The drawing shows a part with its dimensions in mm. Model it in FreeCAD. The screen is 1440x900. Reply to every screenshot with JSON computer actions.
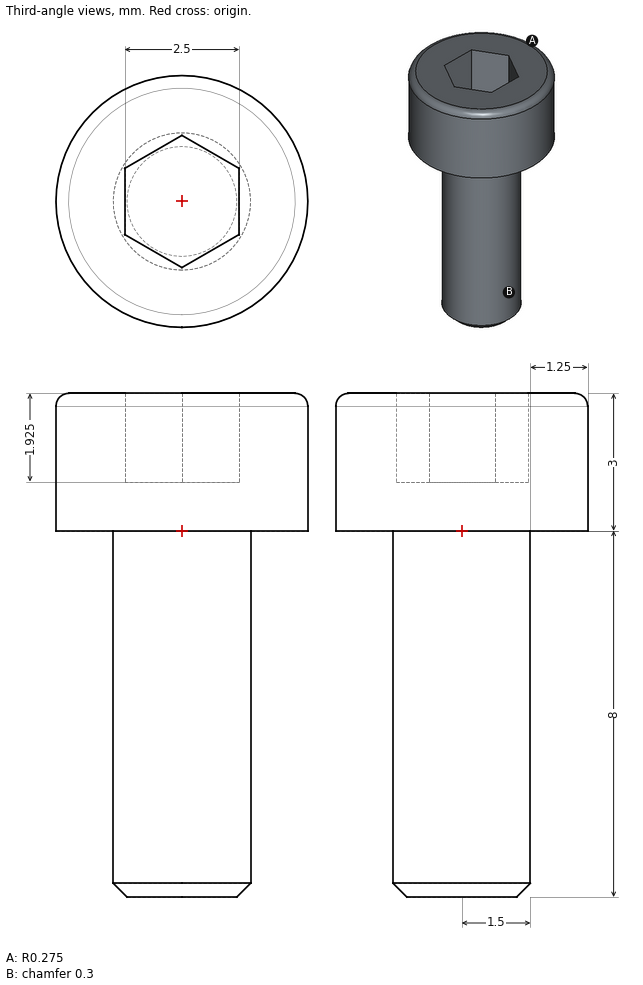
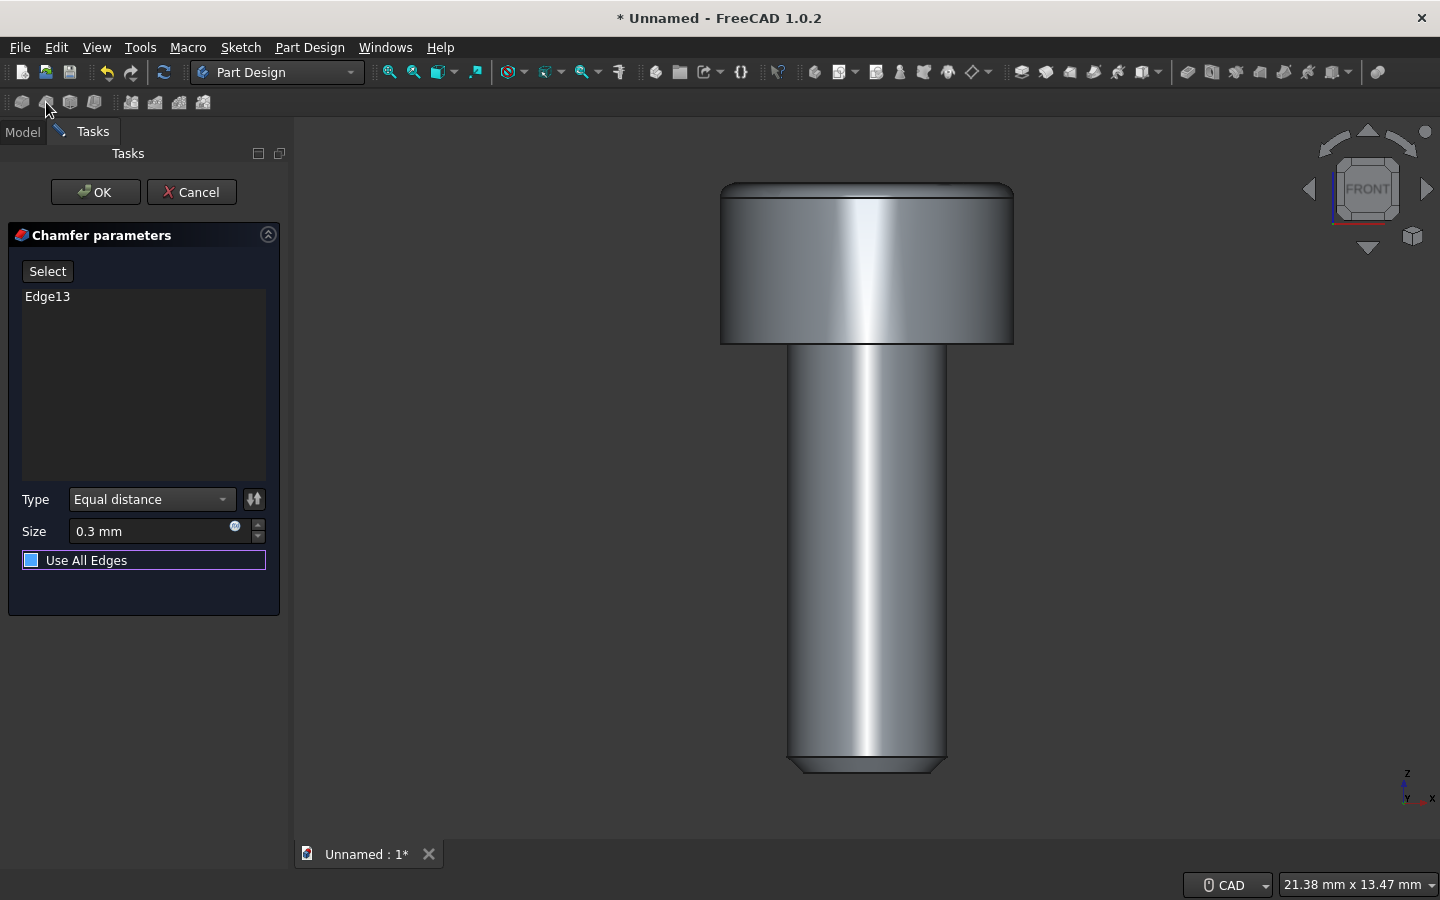
{"action": "left_click", "coordinate": [96, 192]}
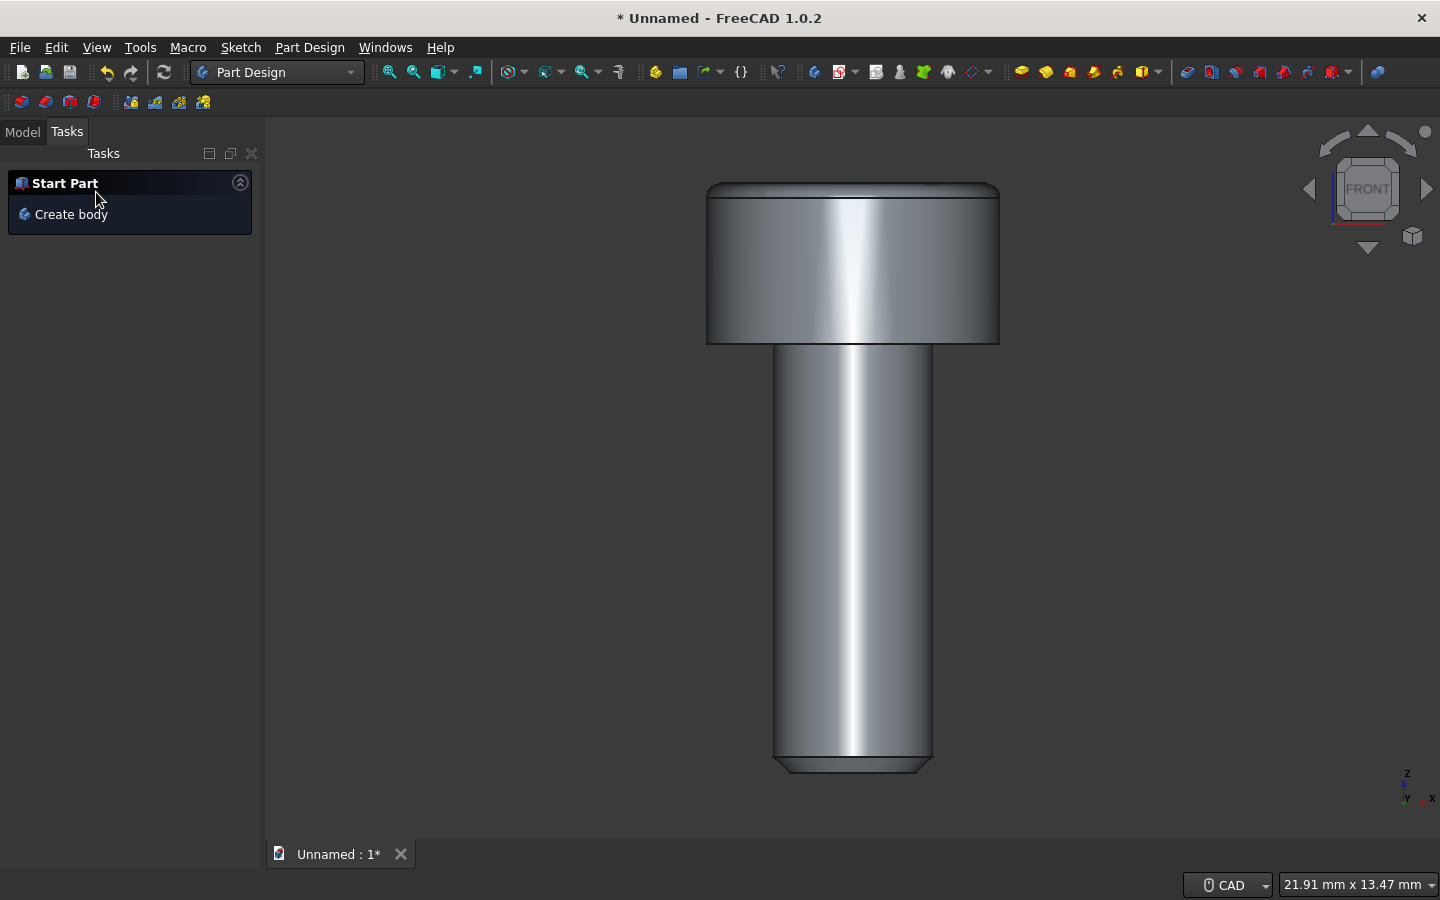
{"action": "key", "text": "0"}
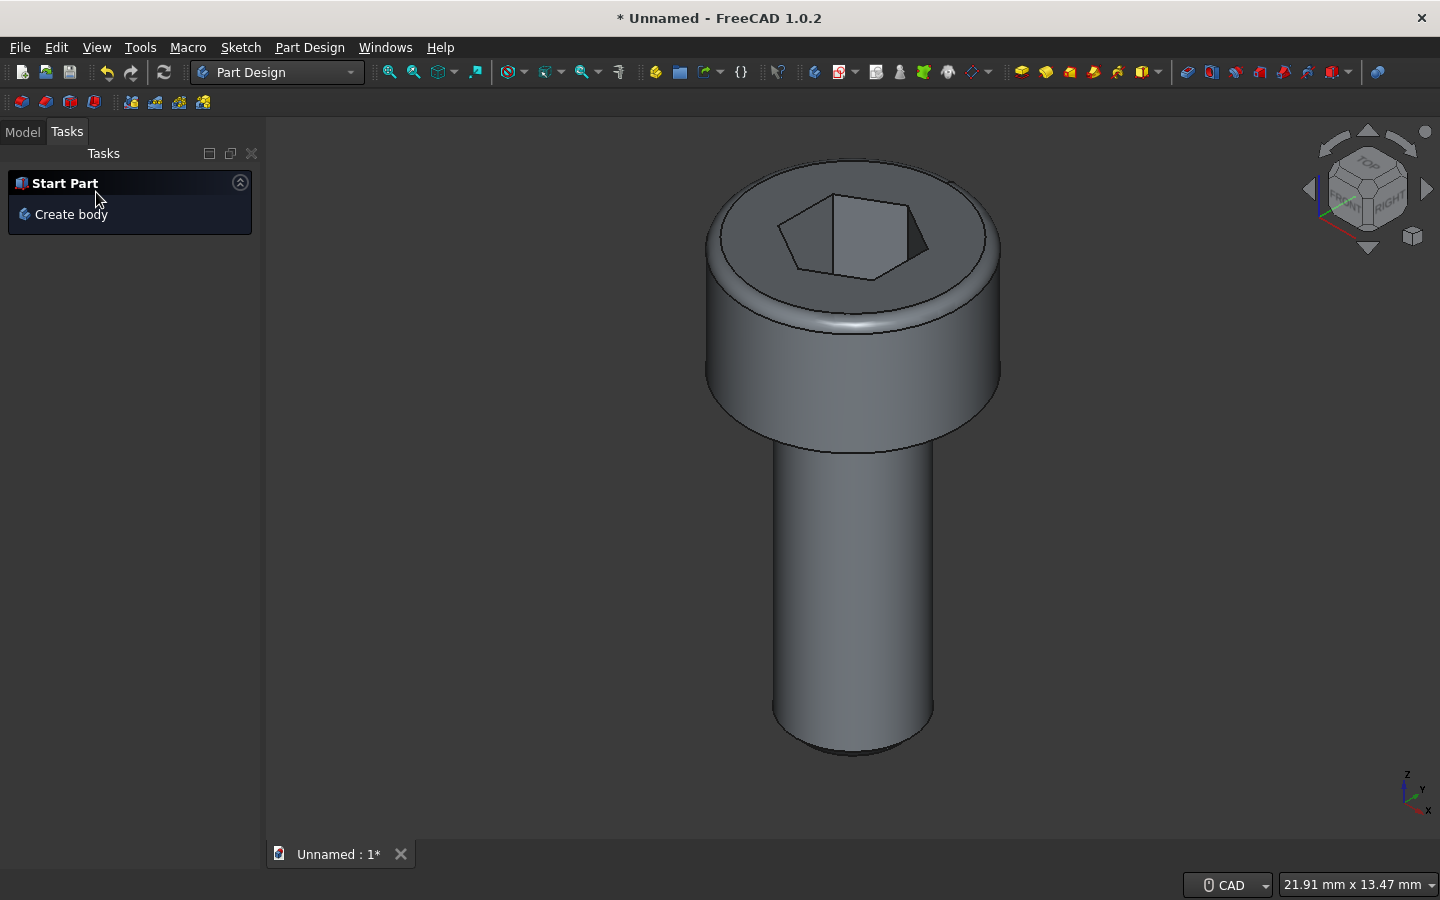
{"action": "left_click", "coordinate": [390, 72]}